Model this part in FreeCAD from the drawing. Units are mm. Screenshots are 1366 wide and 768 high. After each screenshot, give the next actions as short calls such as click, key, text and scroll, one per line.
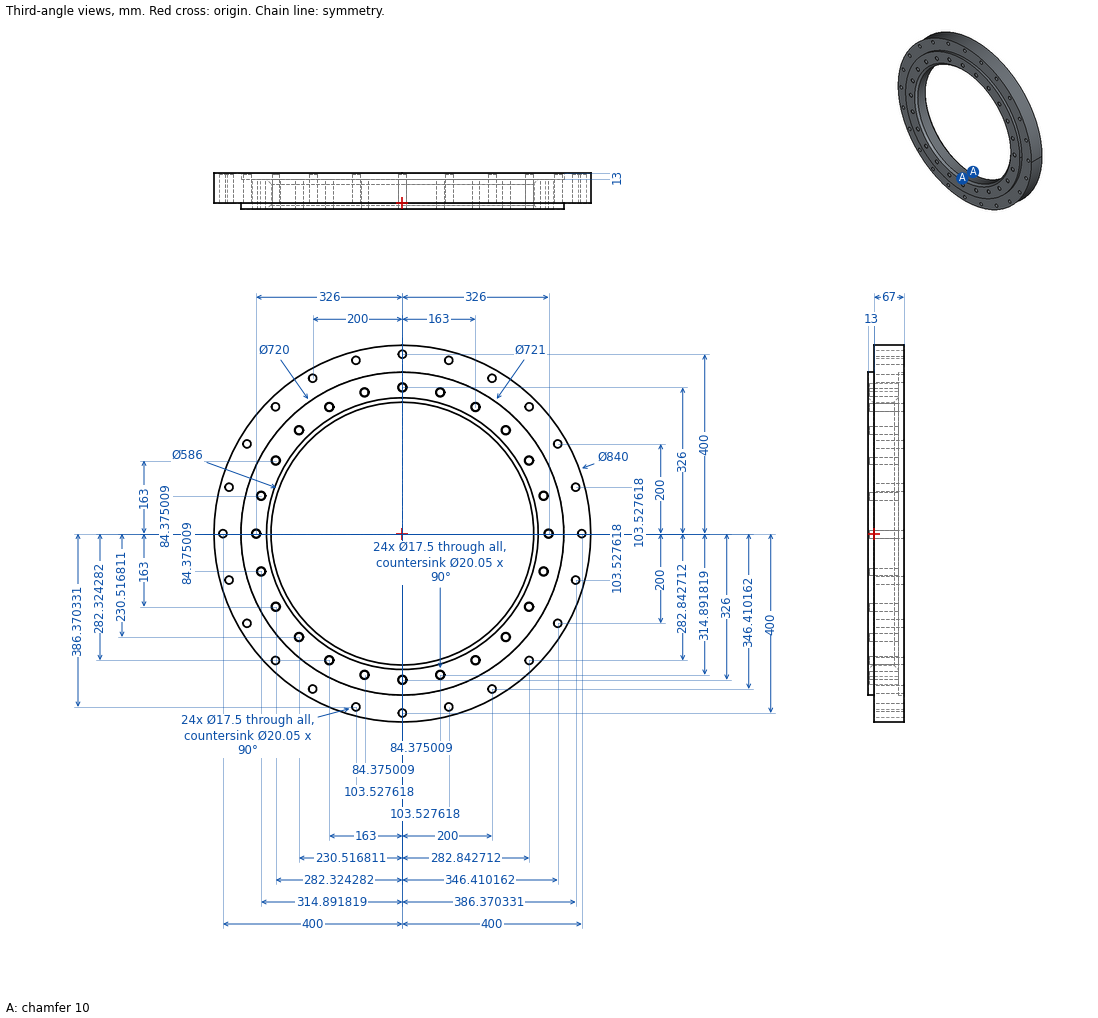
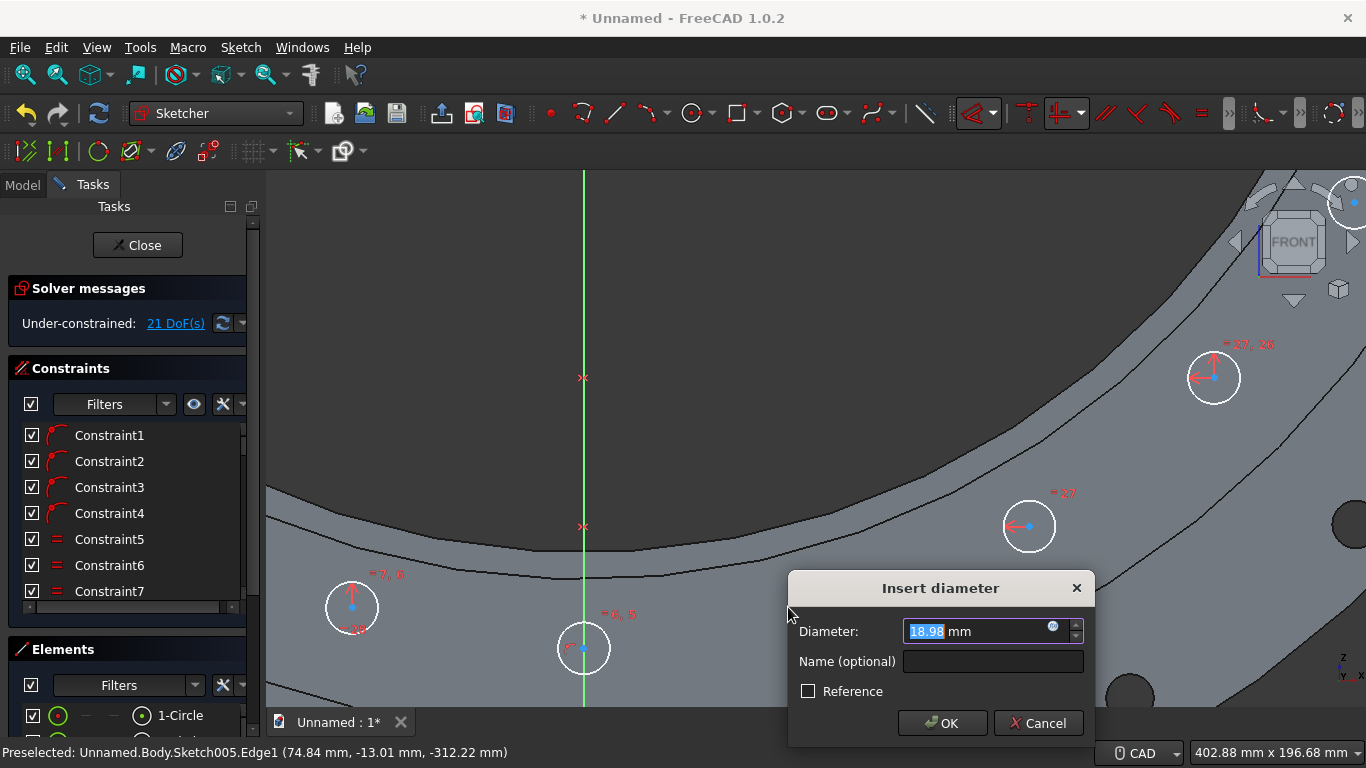
text(17.5)
key(Return)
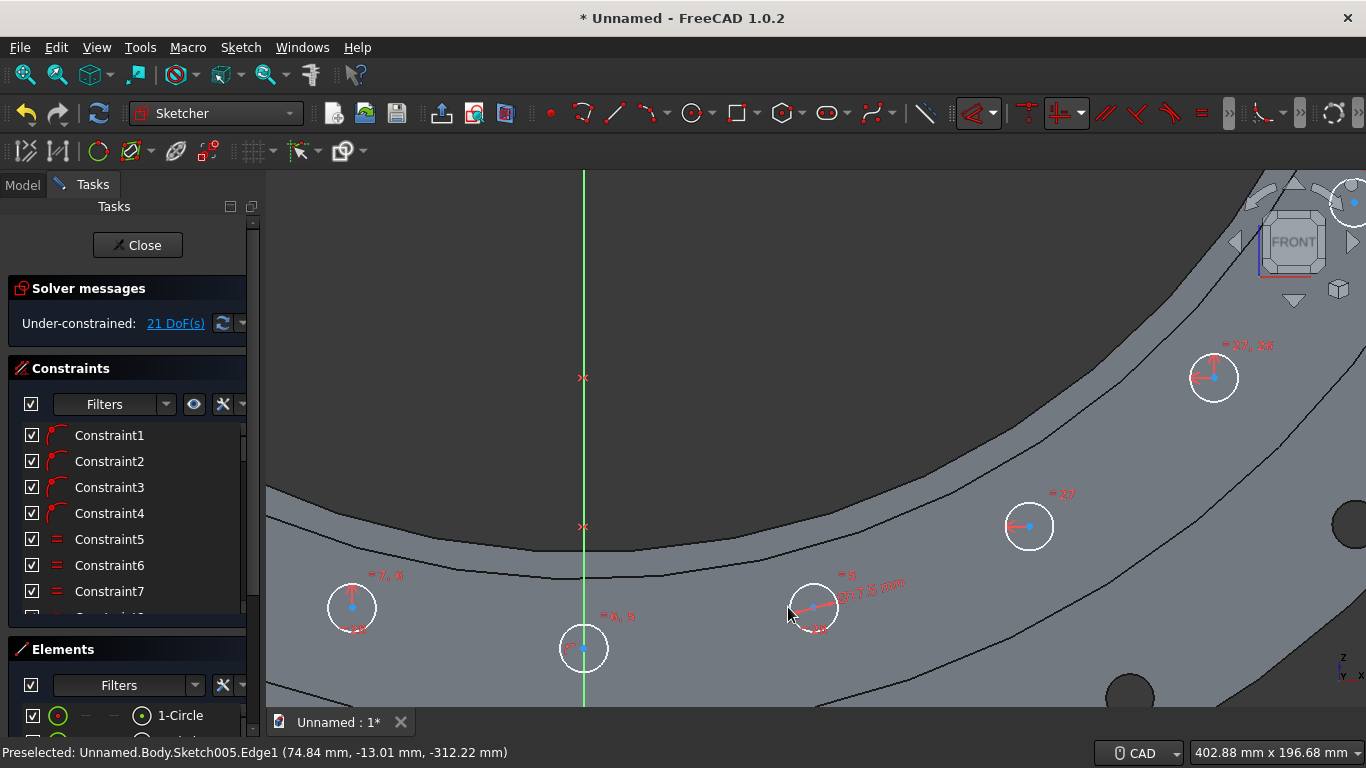
scroll(789, 612, down, 8)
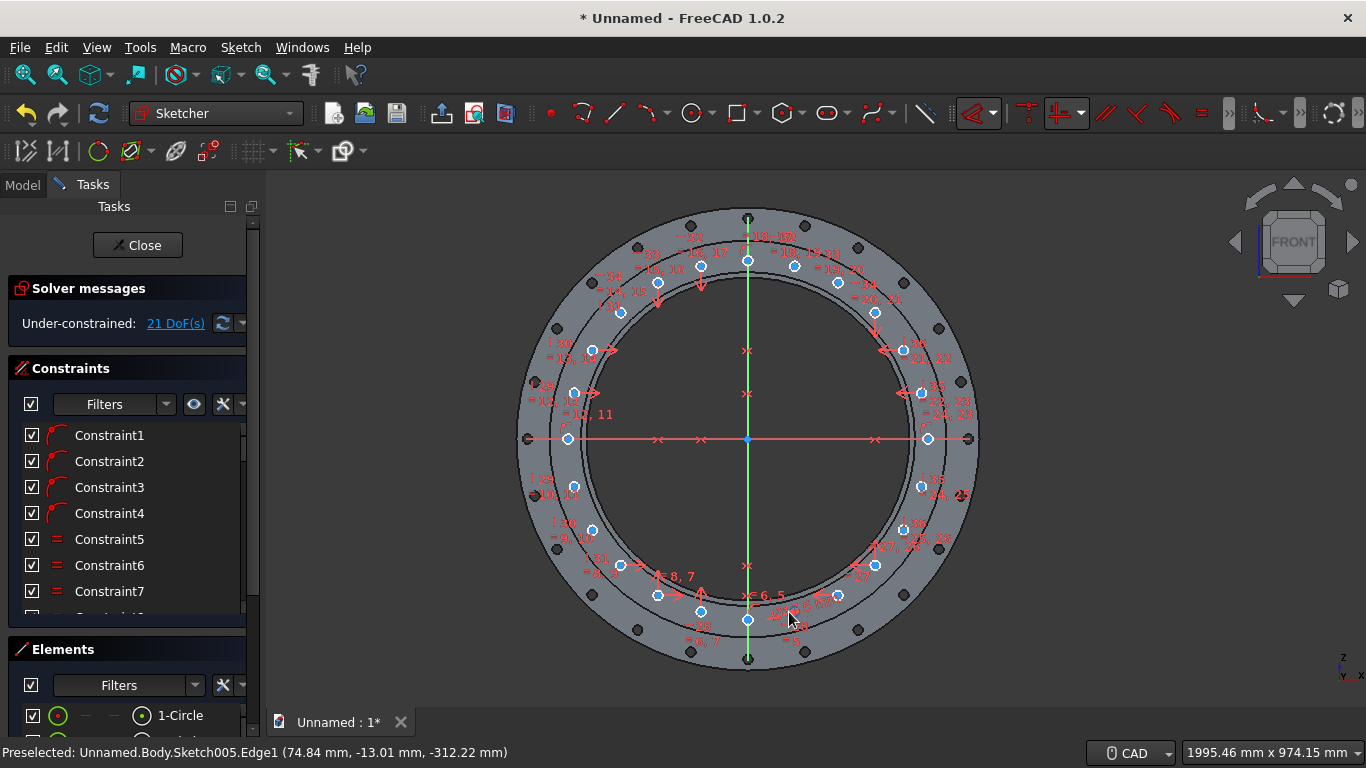
click(748, 620)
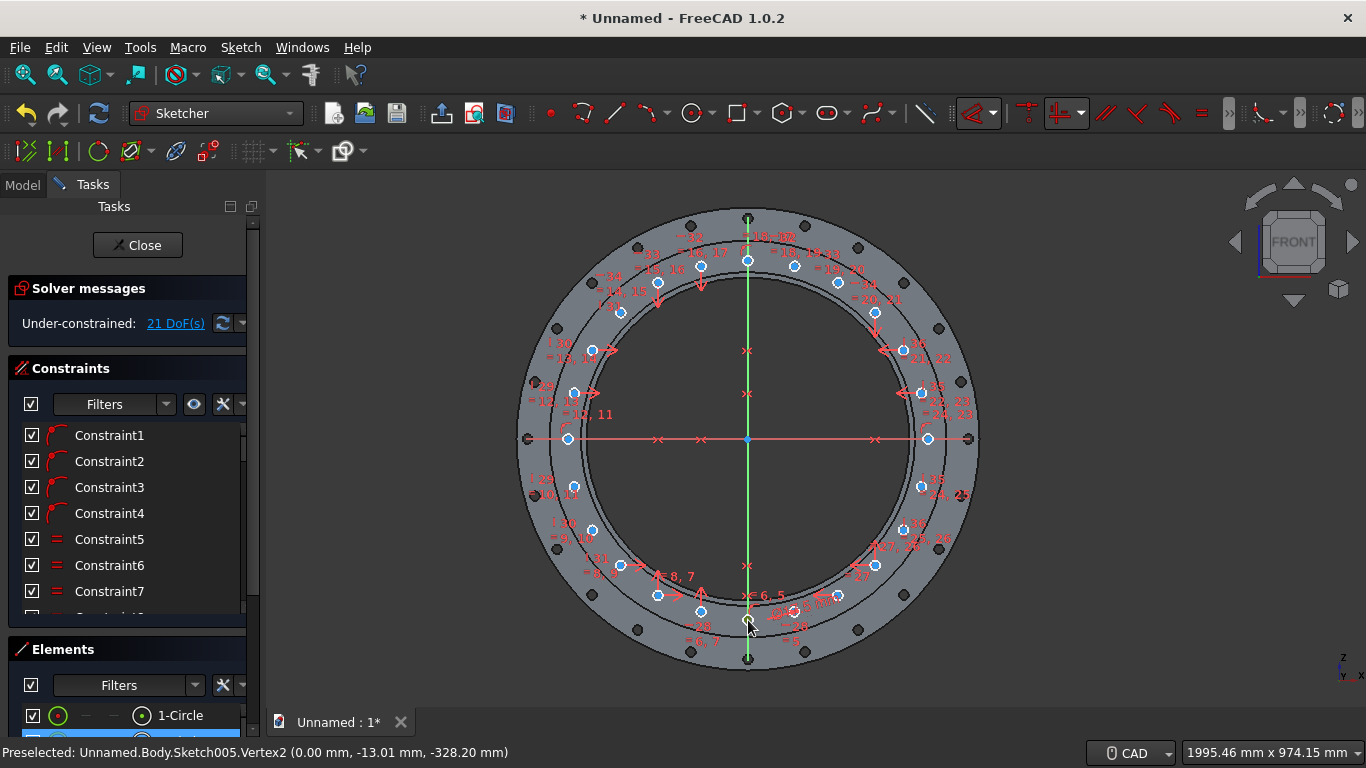
click(996, 114)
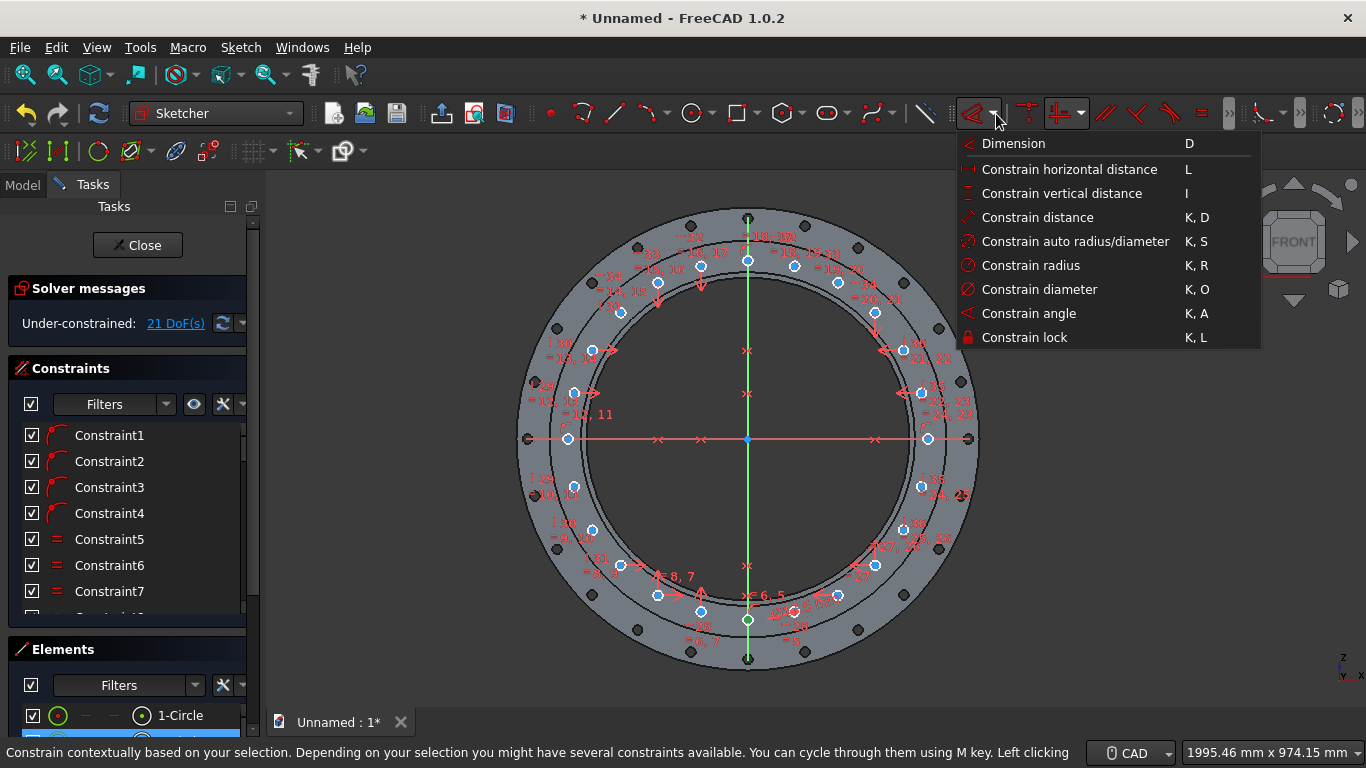
click(1109, 193)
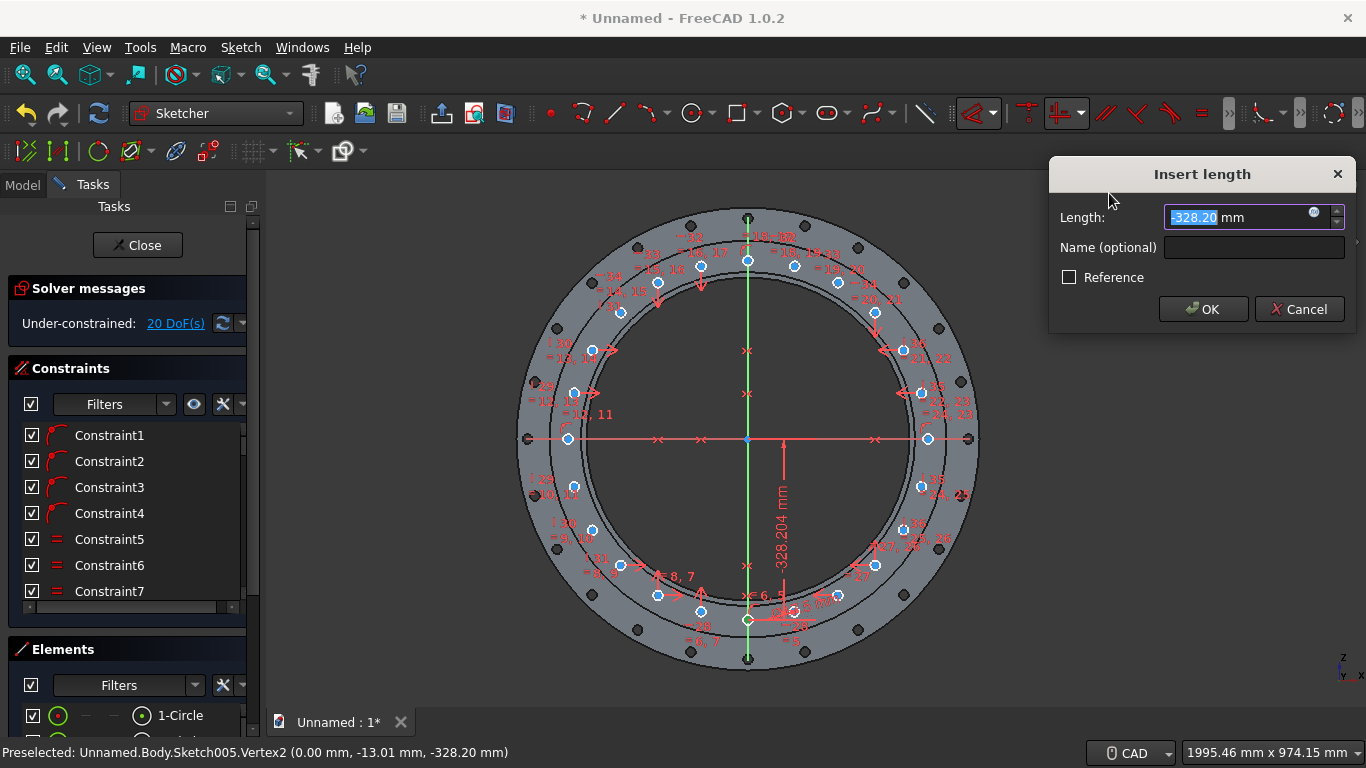
text(-326)
key(Return)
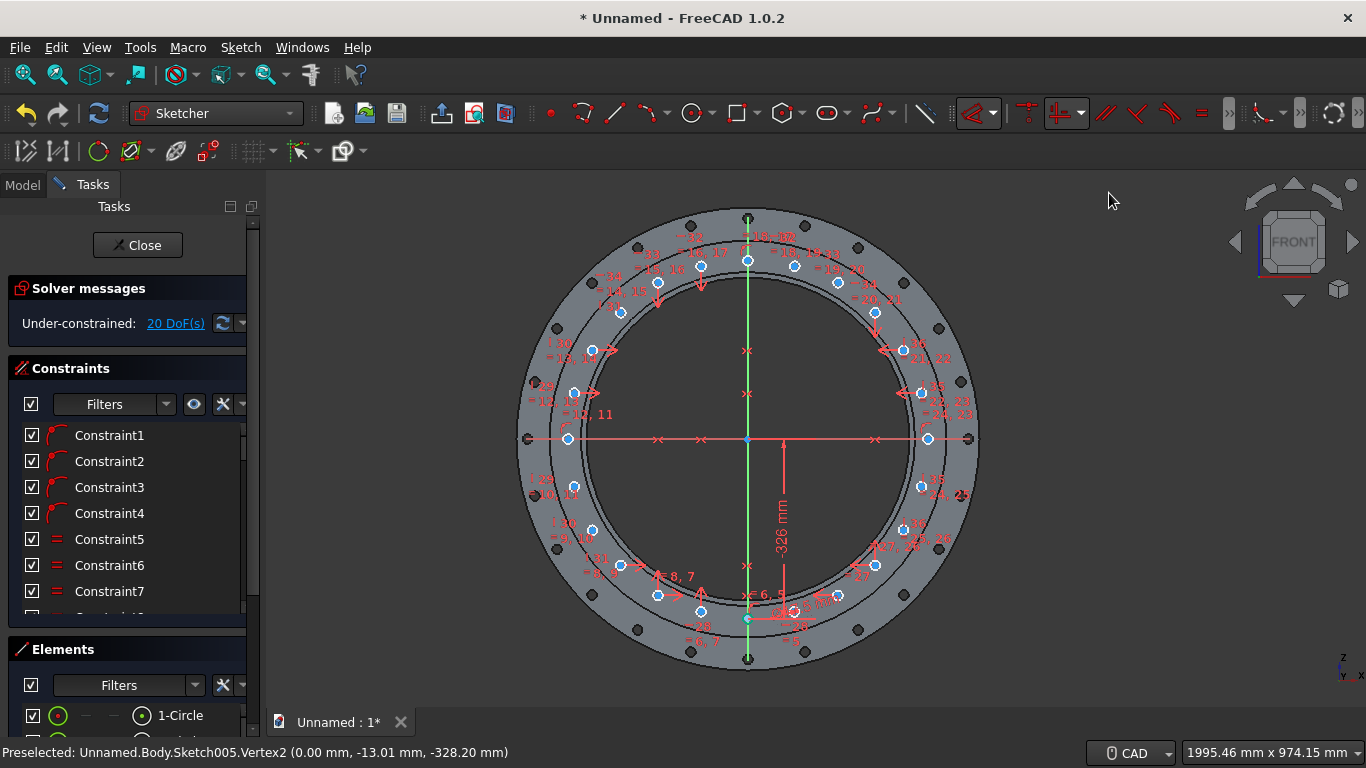
click(658, 595)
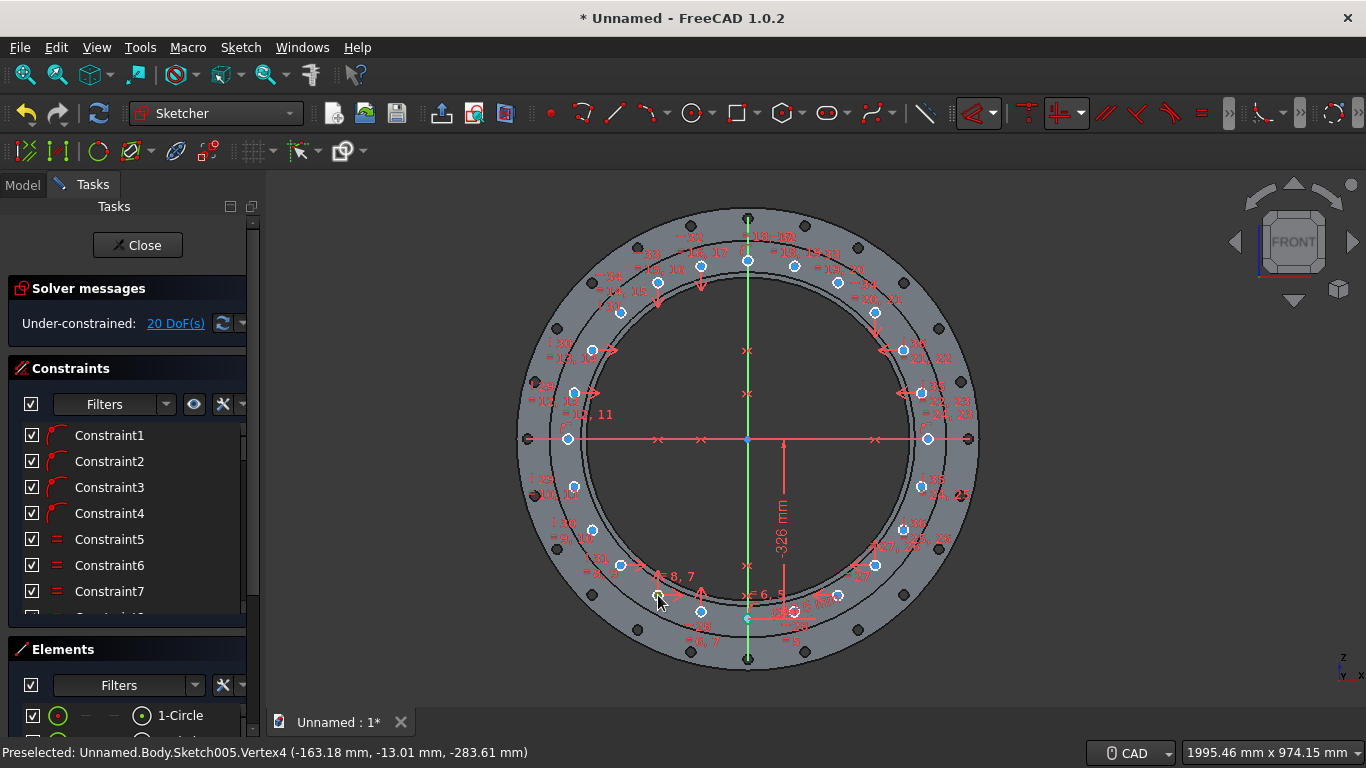
click(996, 114)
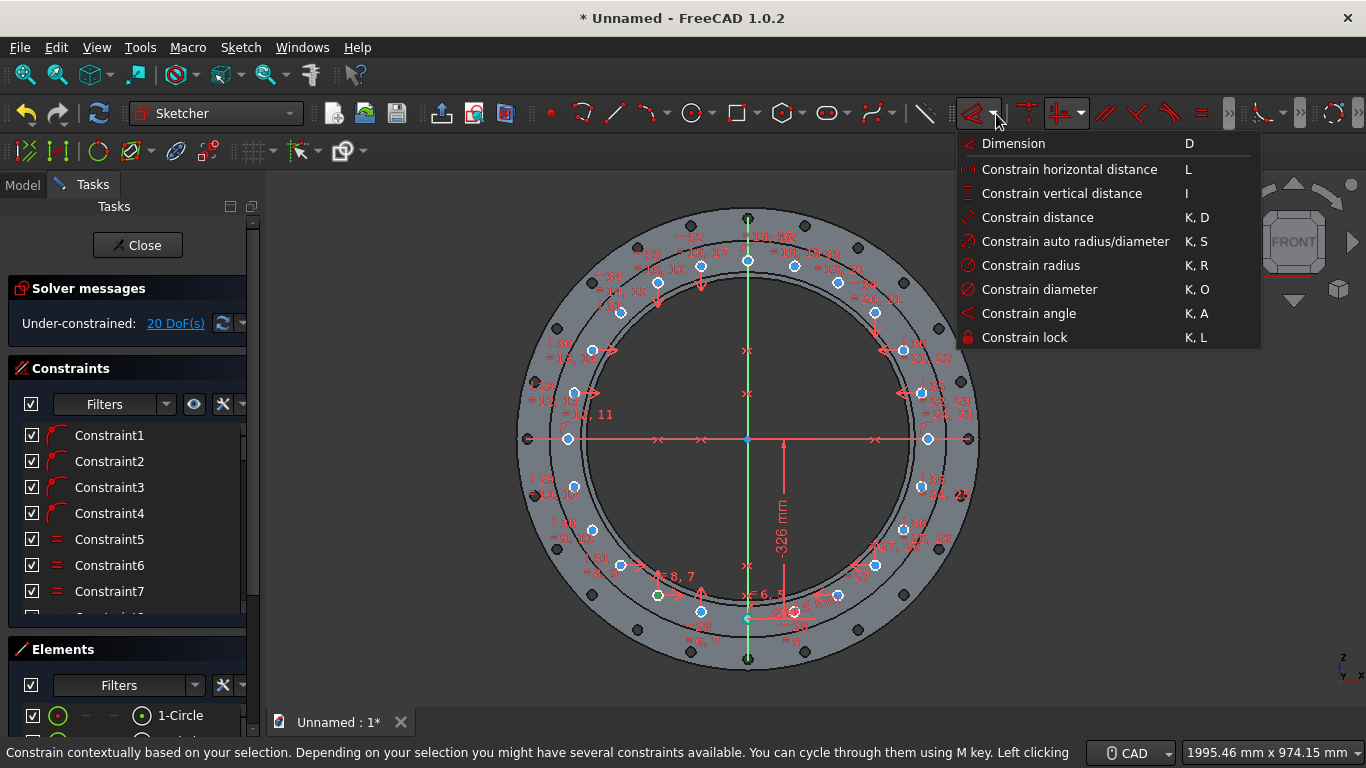
click(1109, 169)